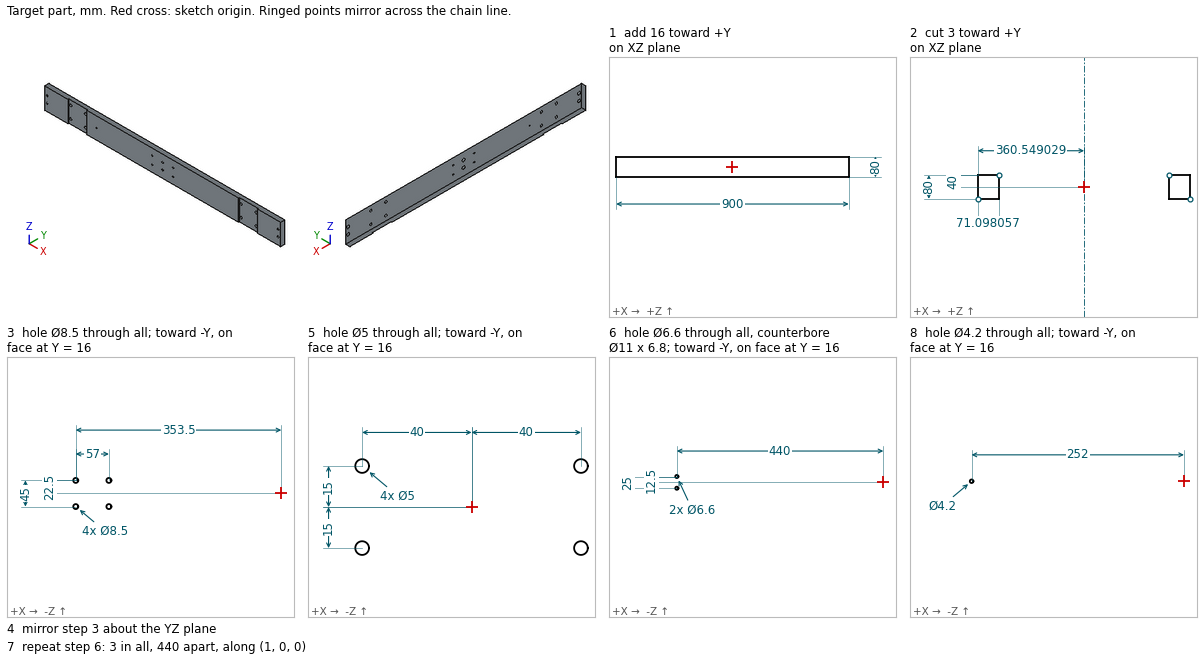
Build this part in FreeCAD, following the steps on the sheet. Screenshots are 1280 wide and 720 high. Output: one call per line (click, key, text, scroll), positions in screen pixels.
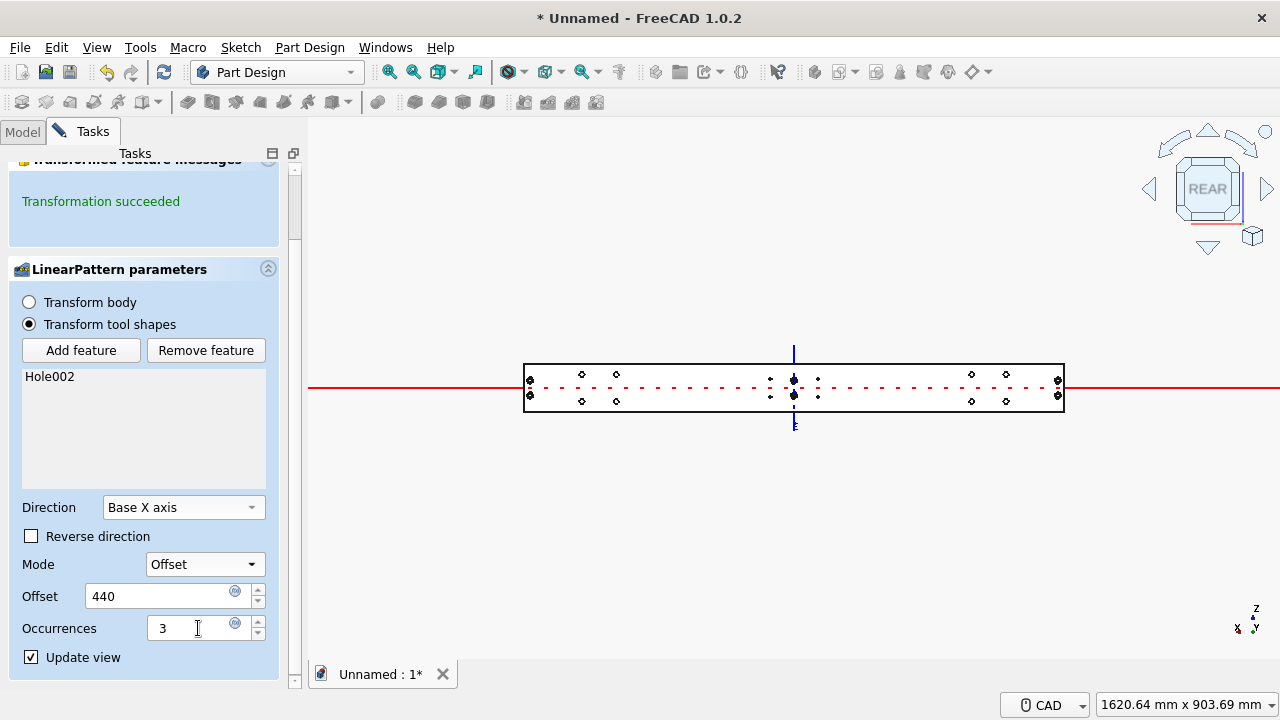
scroll(295, 426, up, 3)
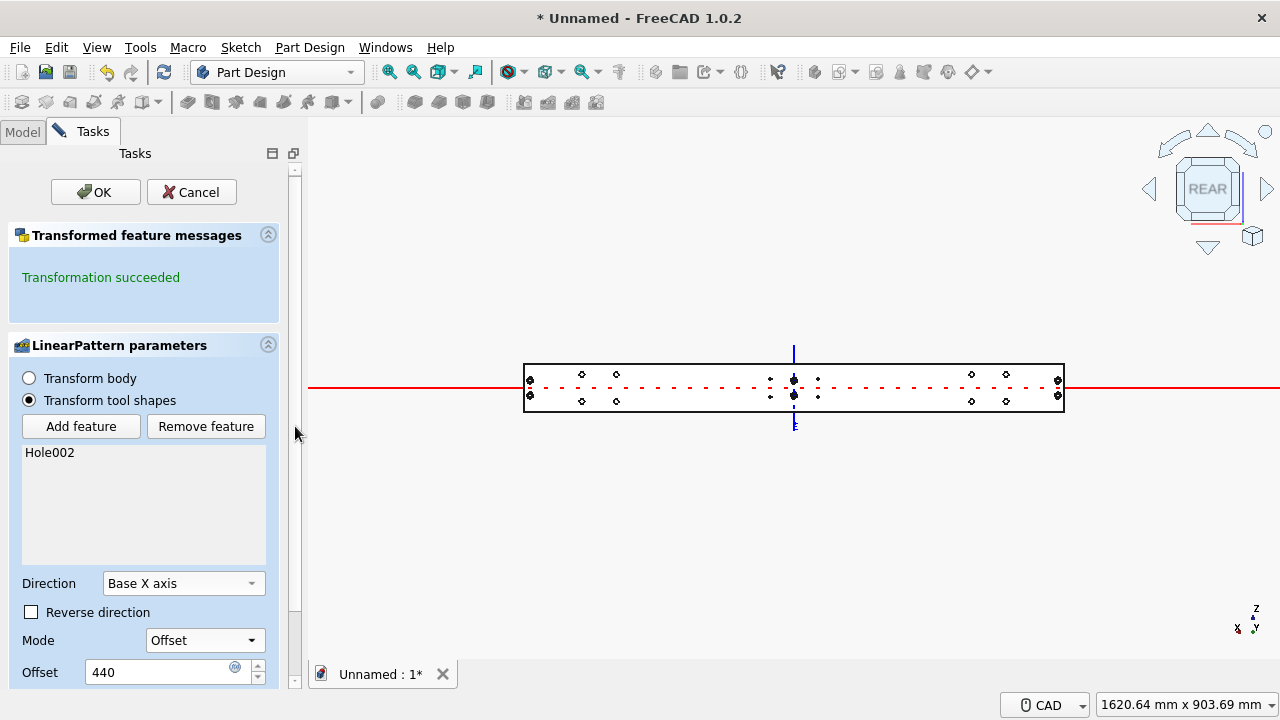
click(96, 192)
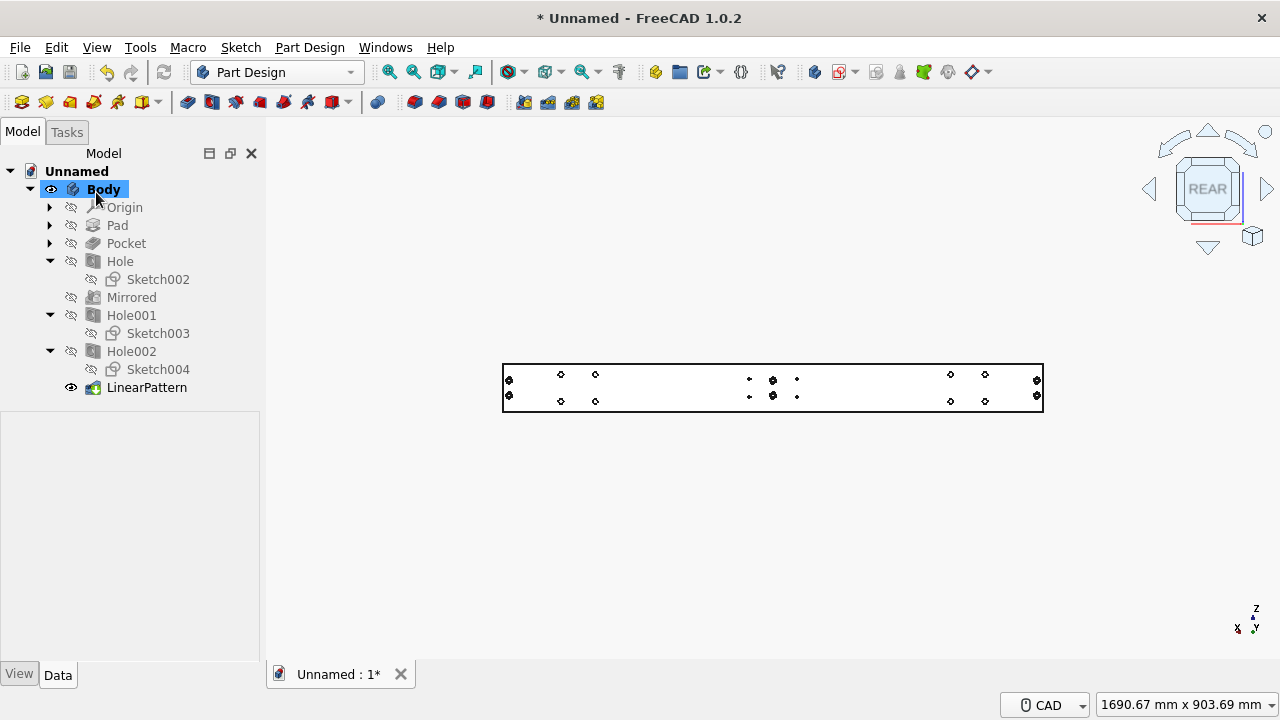
click(619, 387)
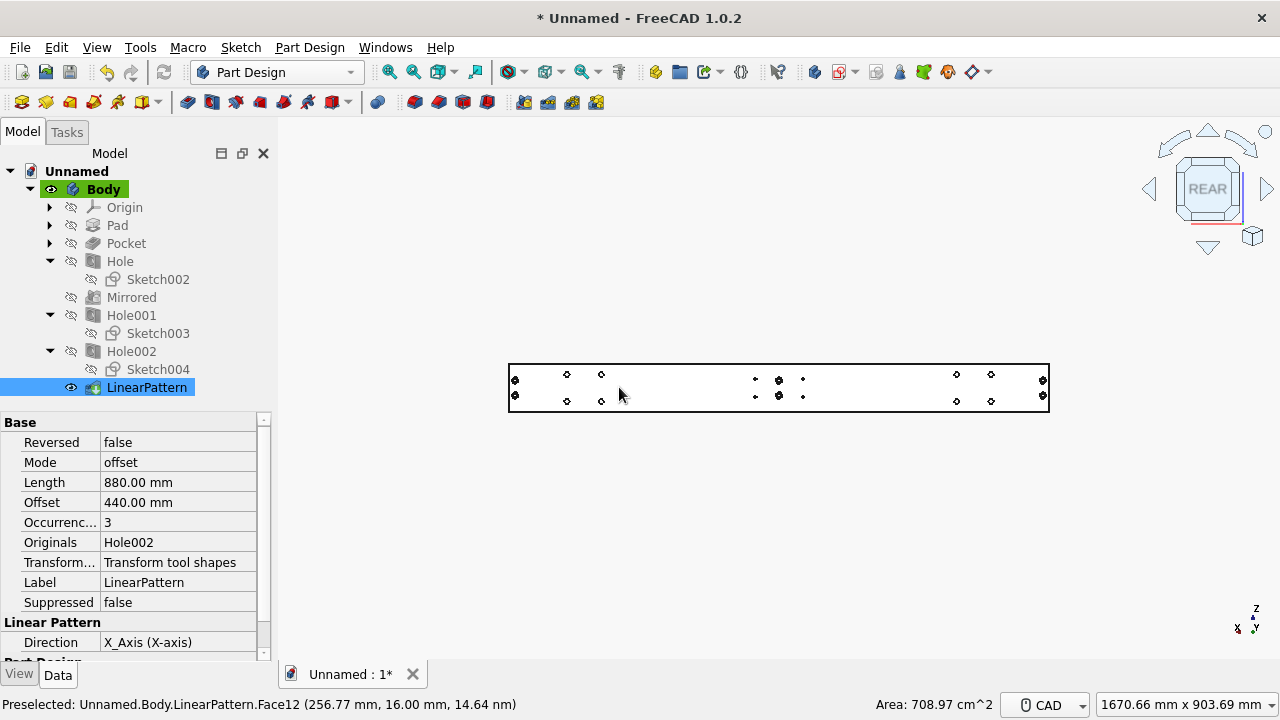
click(840, 72)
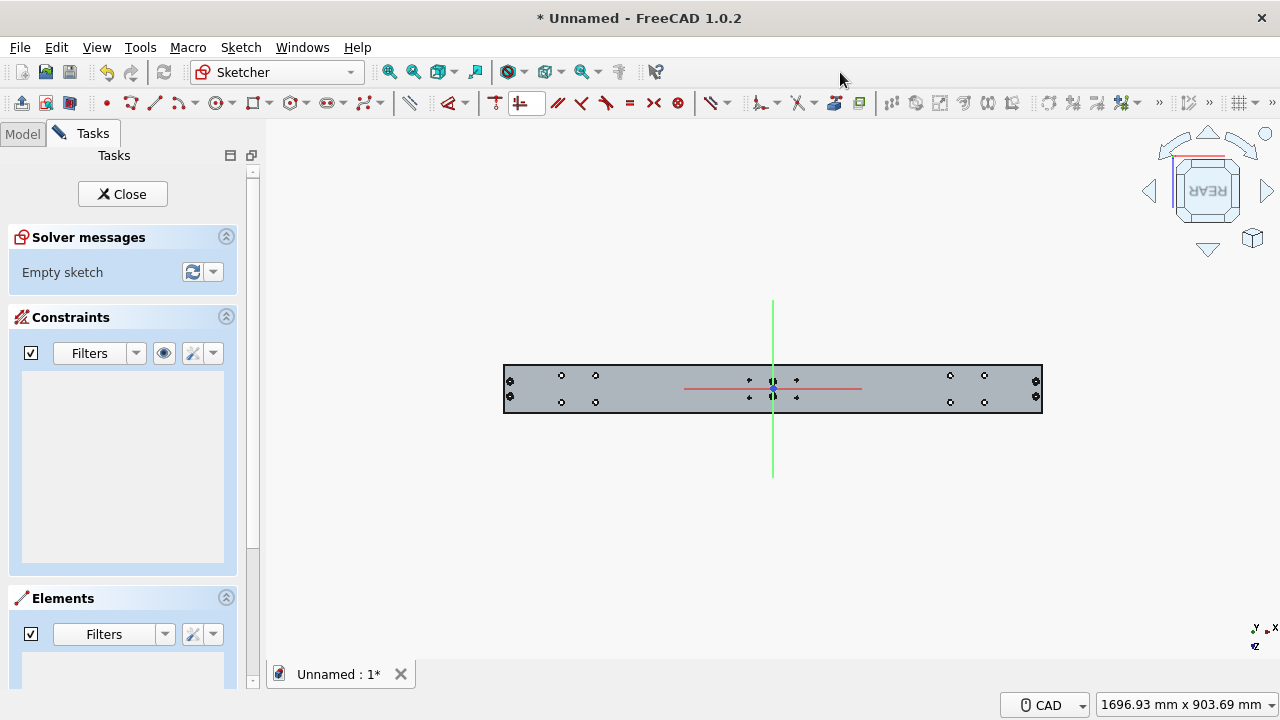
scroll(618, 389, up, 15)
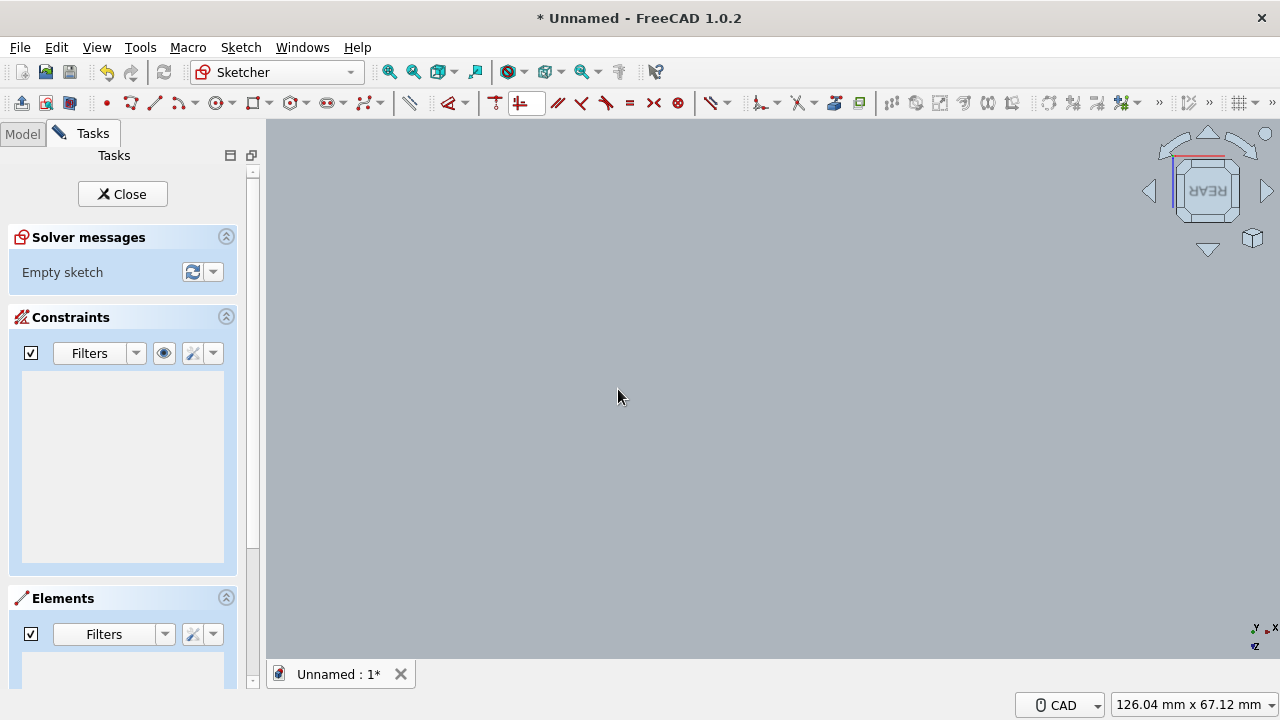
scroll(699, 378, up, 10)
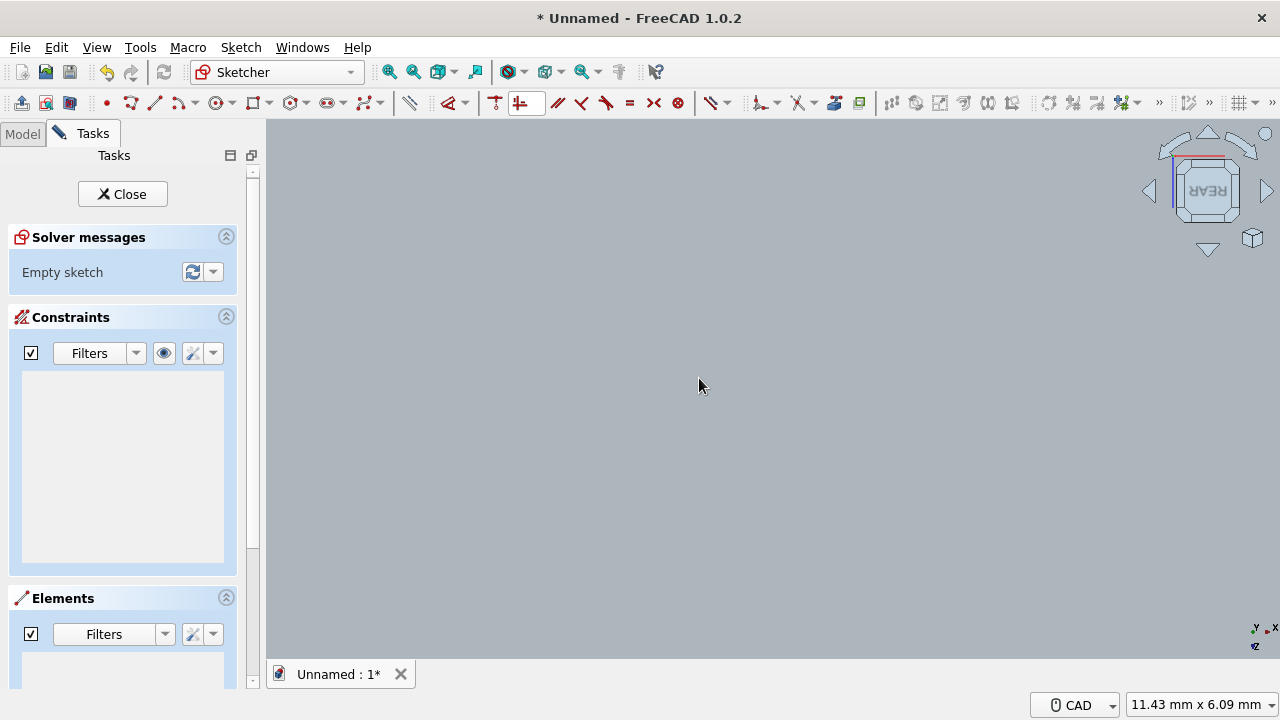
click(216, 104)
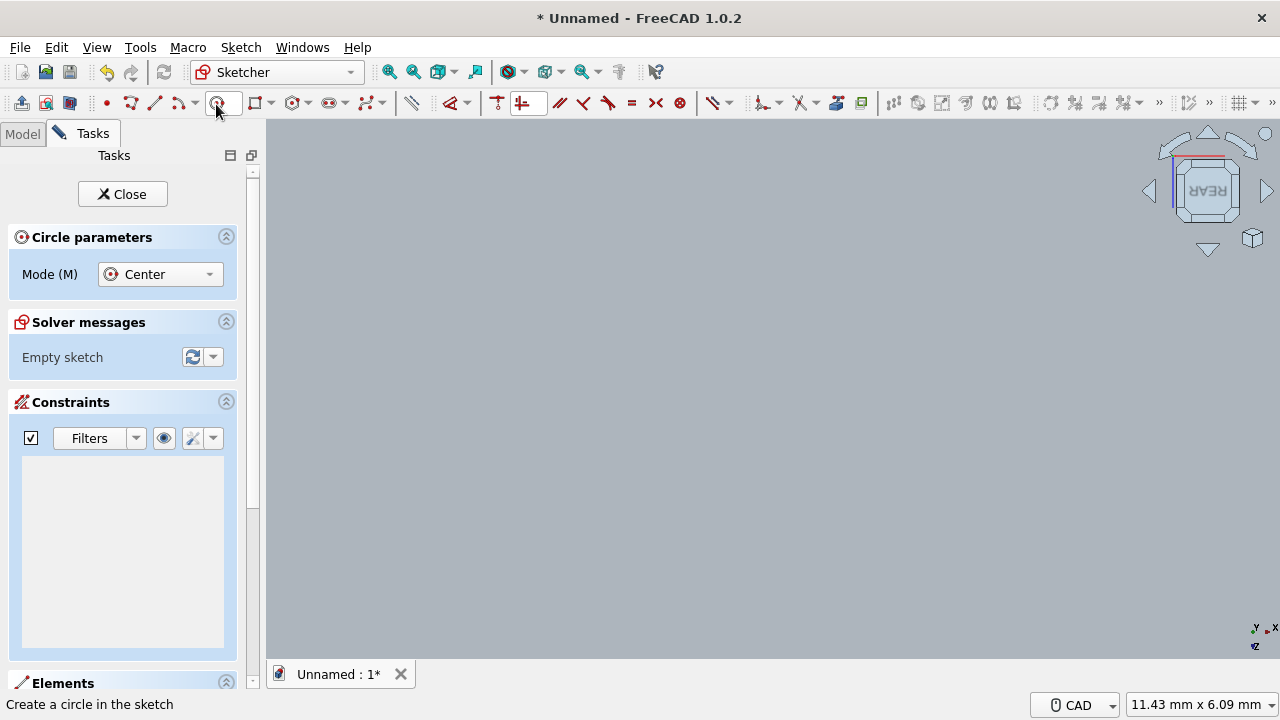
click(704, 386)
click(836, 254)
key(Escape)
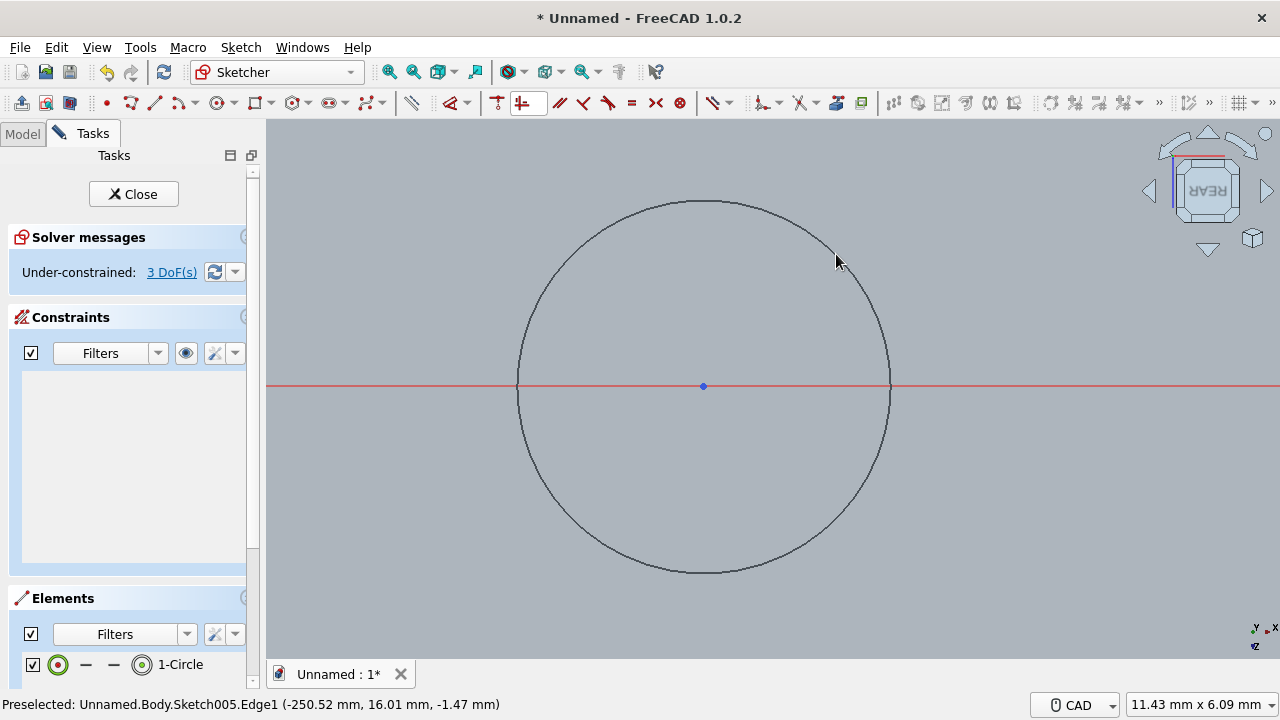
click(704, 387)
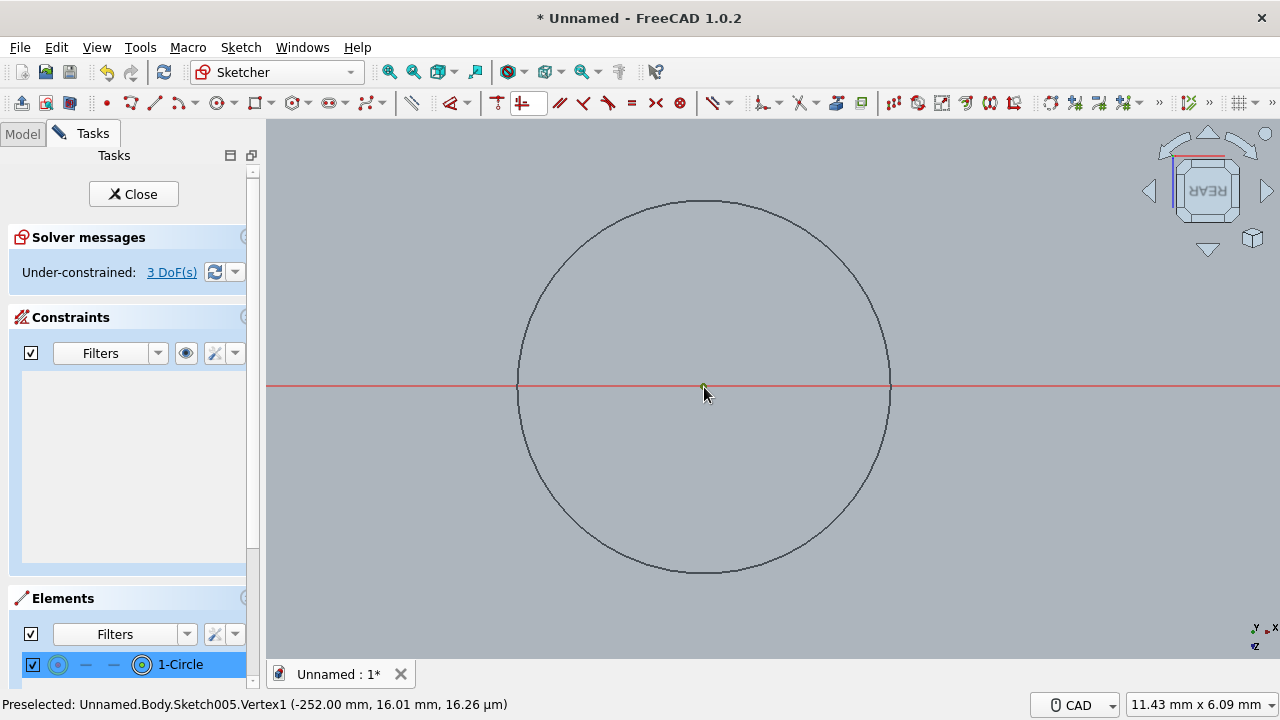
click(353, 386)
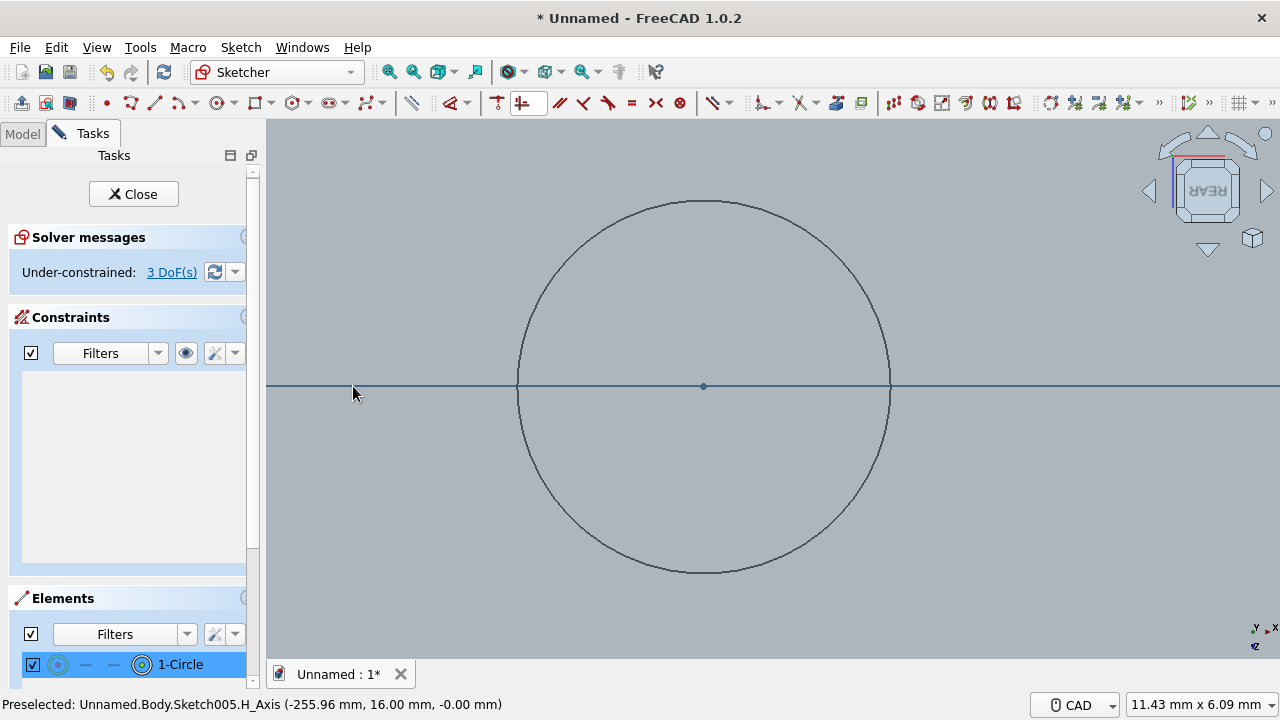
click(498, 104)